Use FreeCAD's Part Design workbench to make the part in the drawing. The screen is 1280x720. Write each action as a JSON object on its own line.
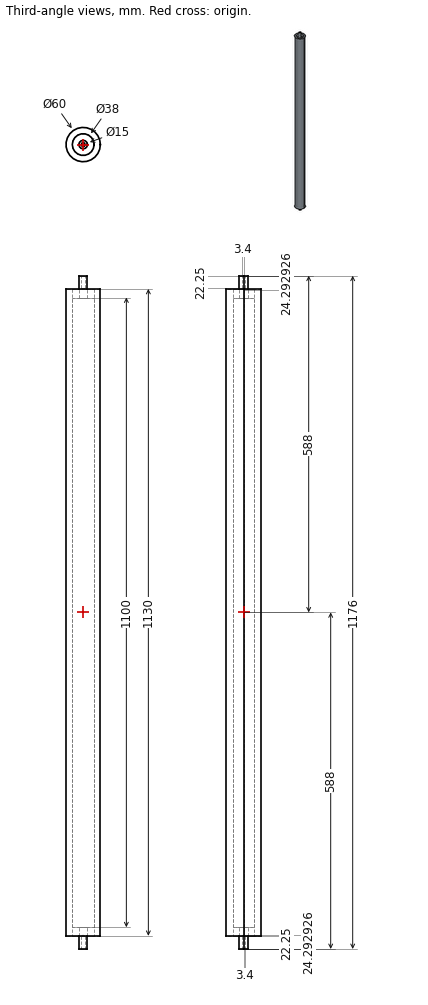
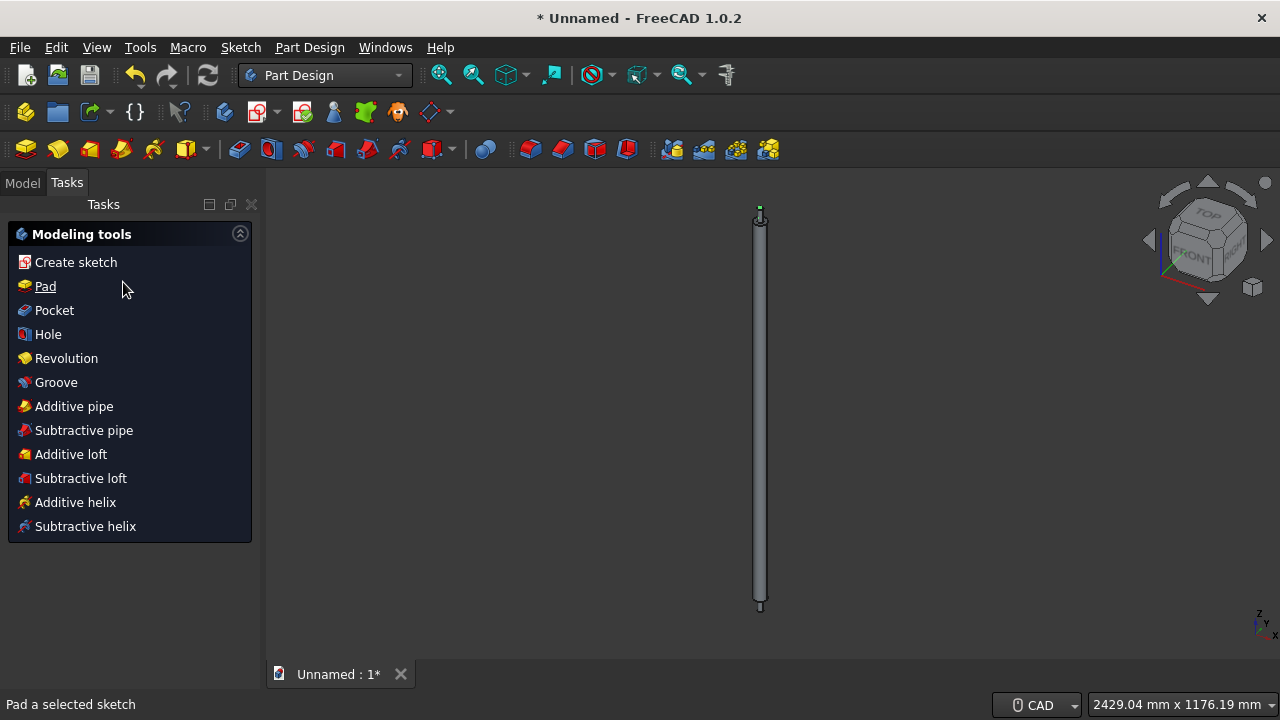
{"action": "left_click", "coordinate": [304, 150]}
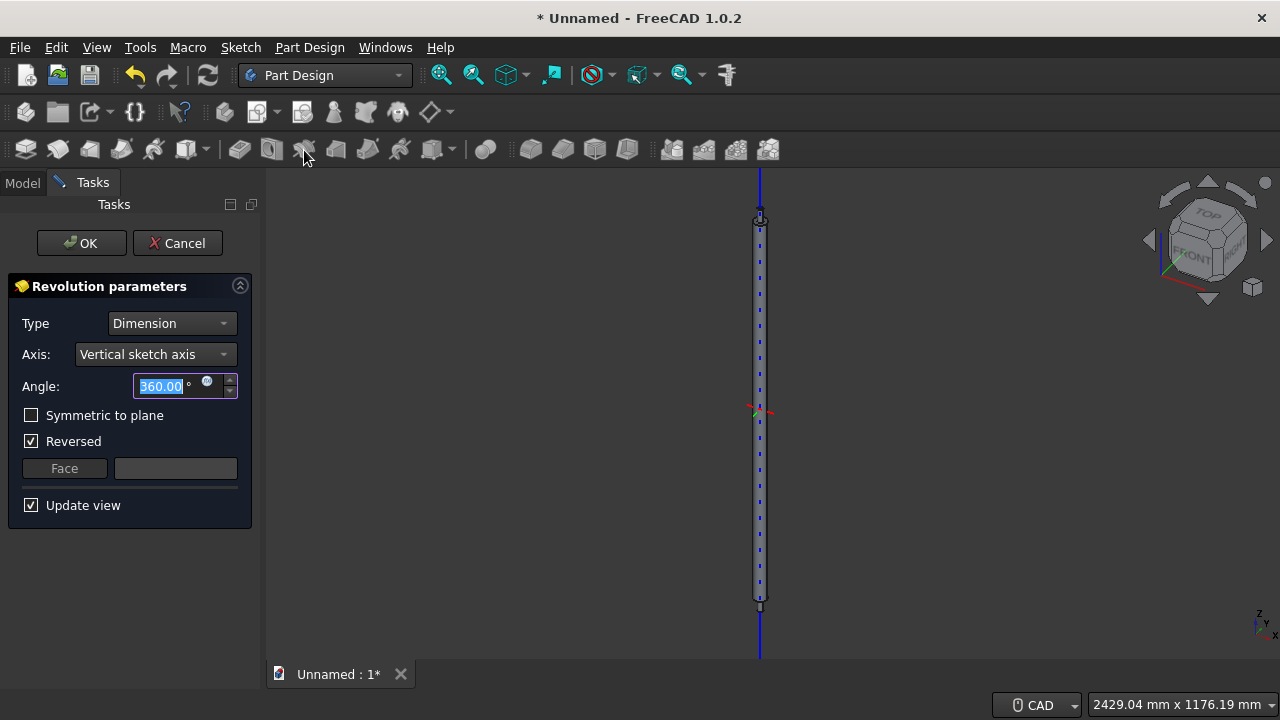
{"action": "left_click", "coordinate": [82, 243]}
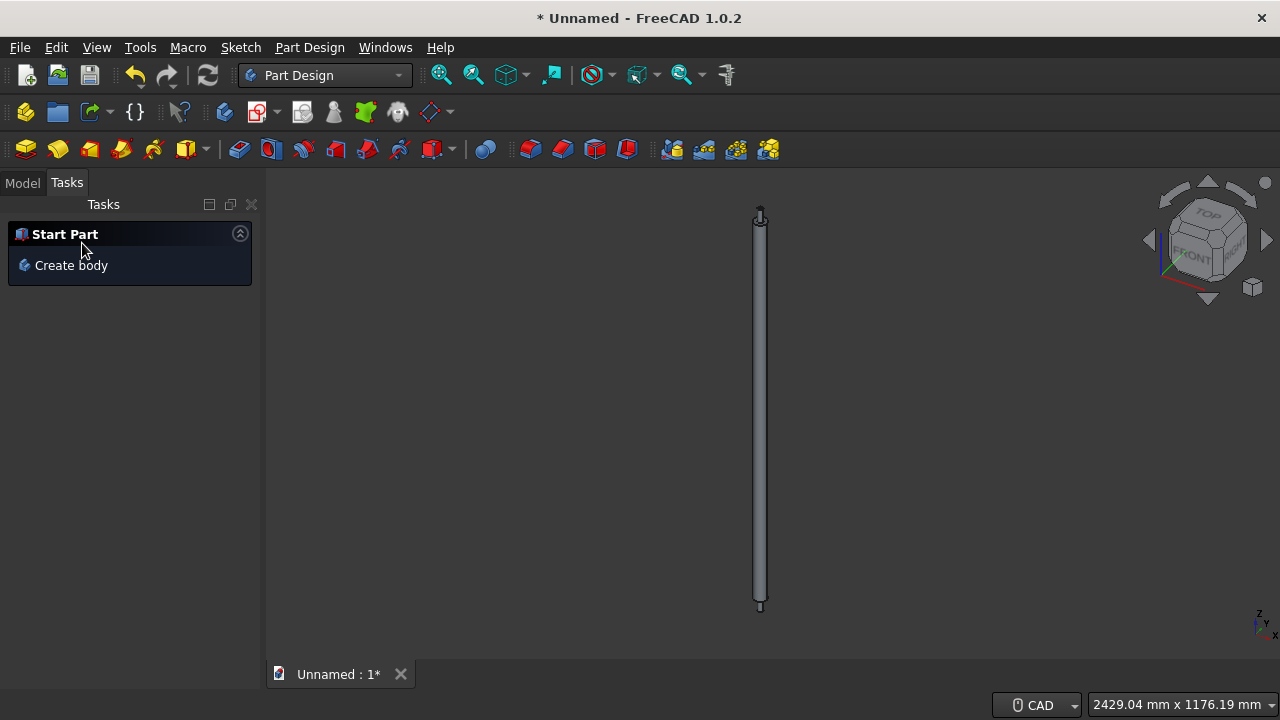
{"action": "left_click", "coordinate": [226, 112]}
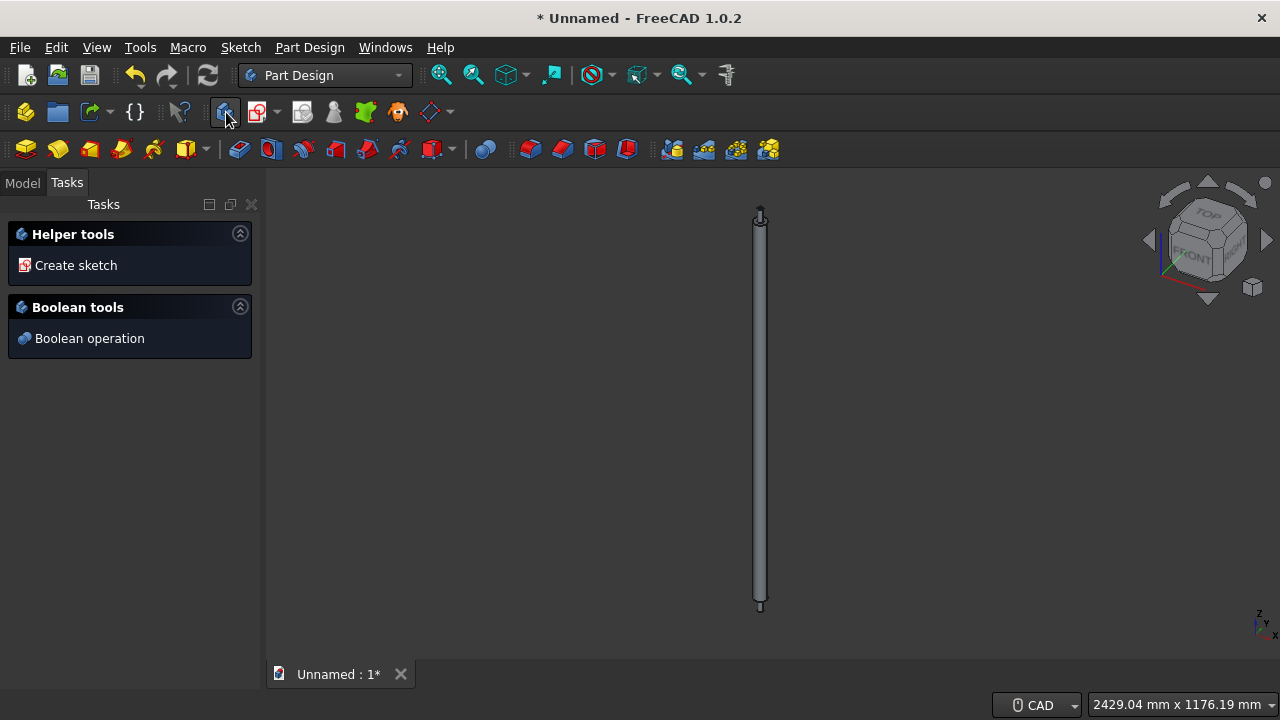
{"action": "left_click", "coordinate": [306, 619]}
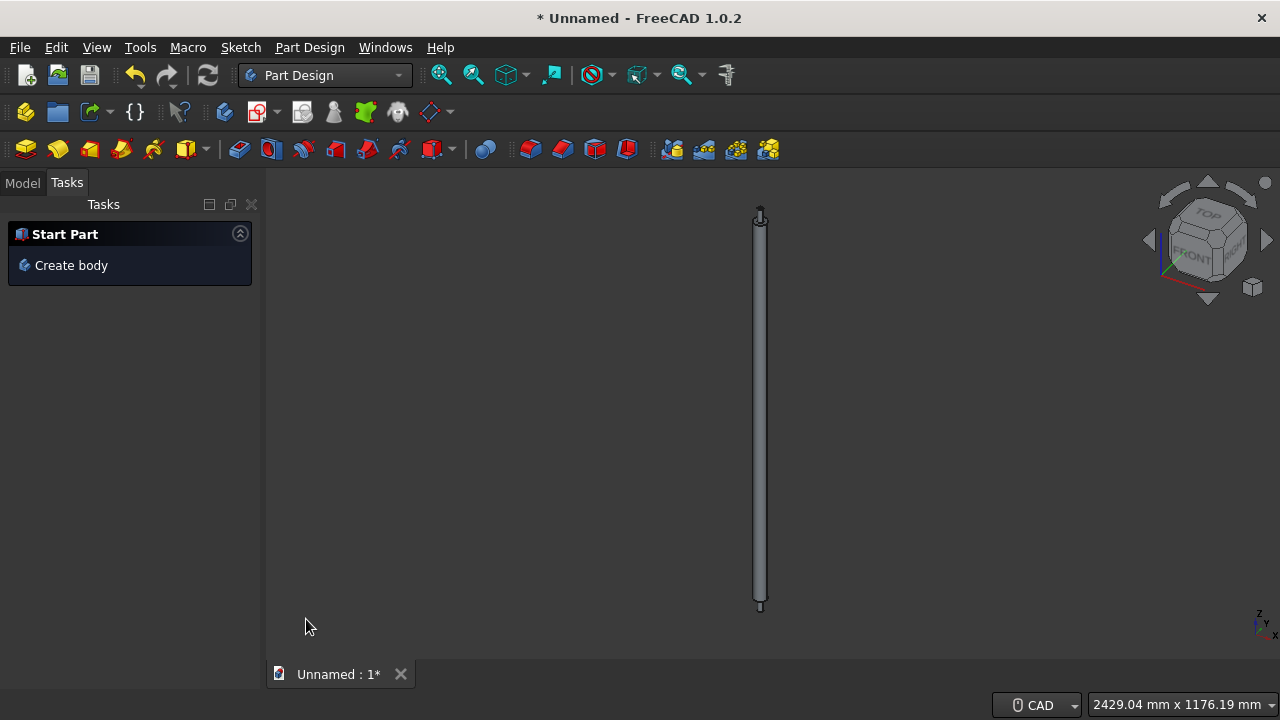
{"action": "left_click", "coordinate": [258, 112]}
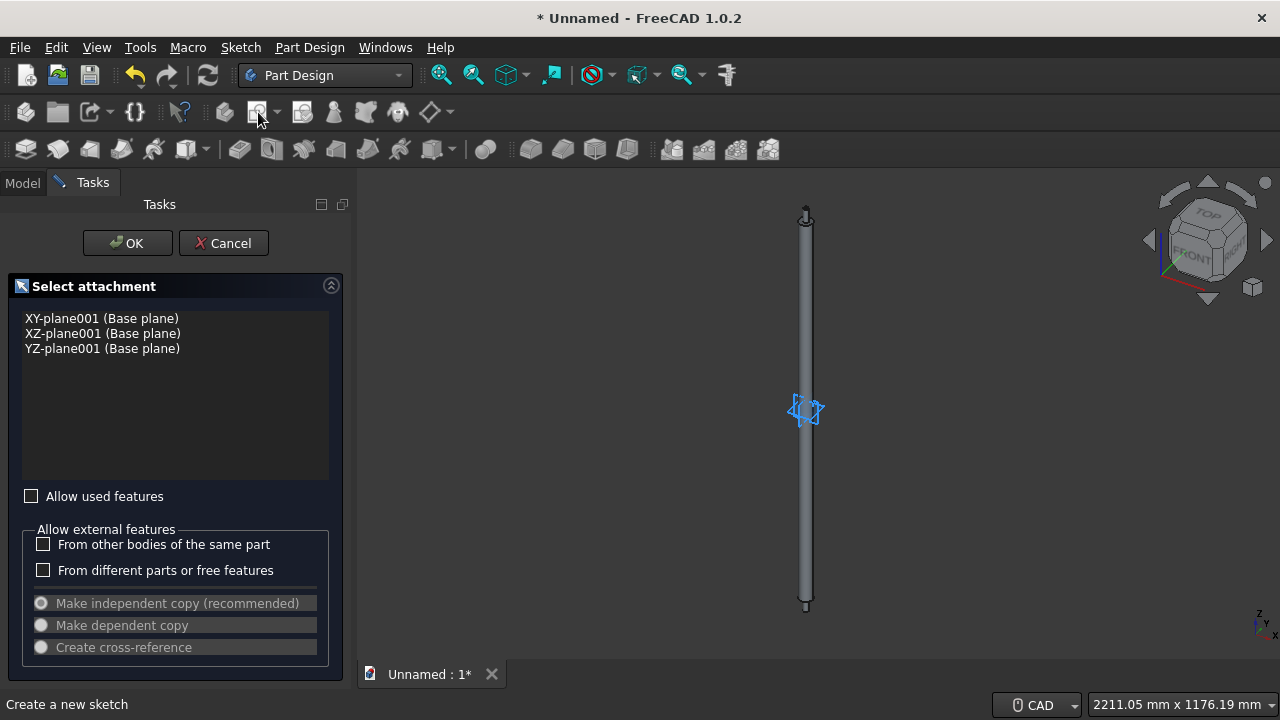
{"action": "left_click", "coordinate": [82, 318]}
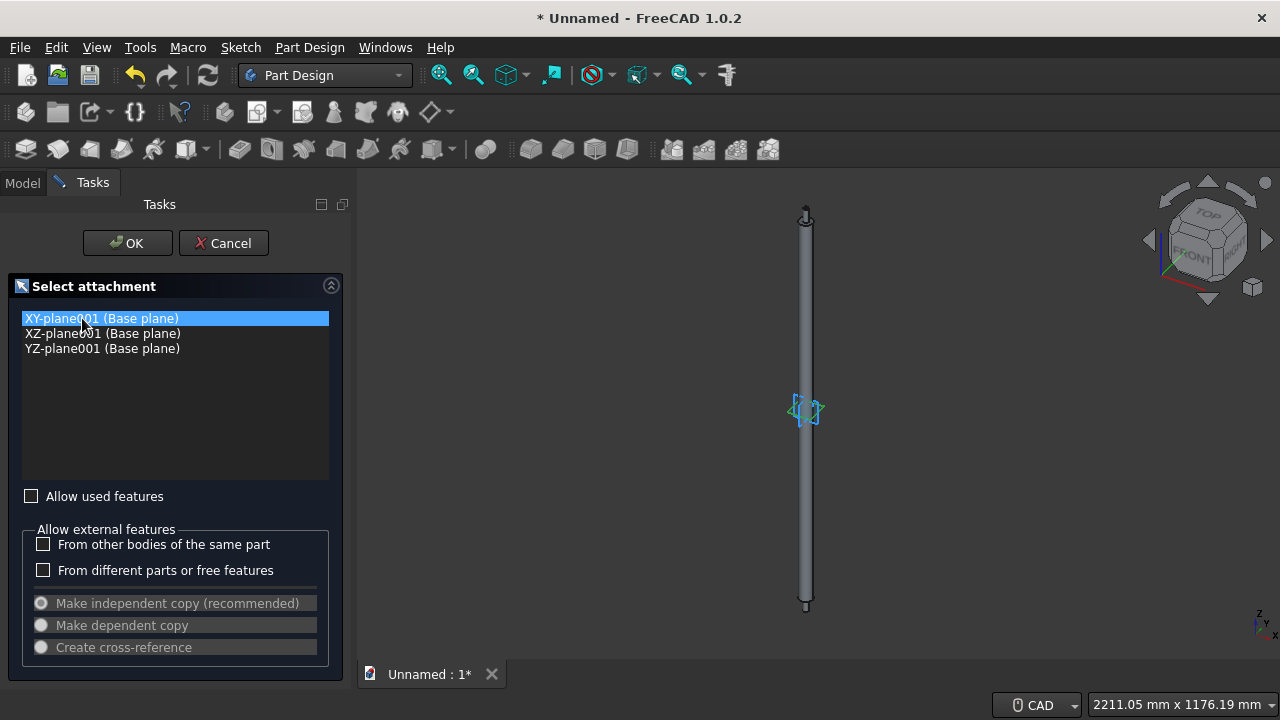
{"action": "left_click", "coordinate": [128, 243]}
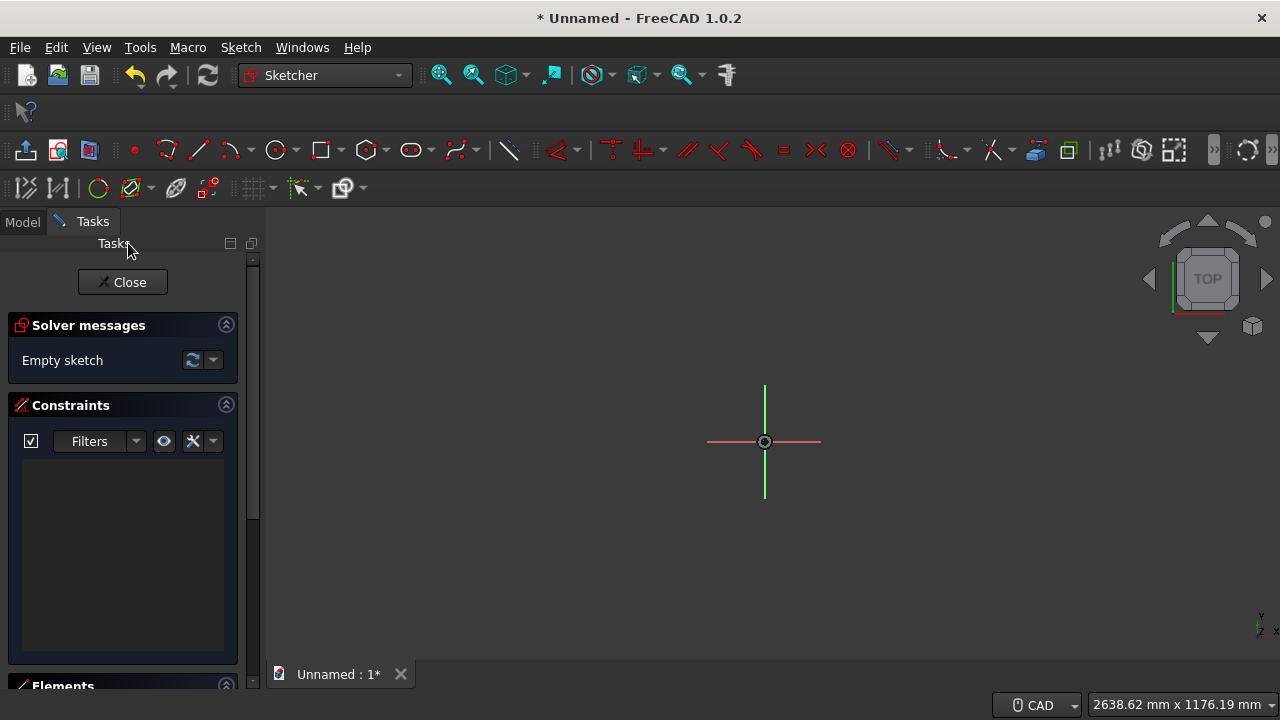
{"action": "scroll", "coordinate": [771, 443], "scroll_direction": "up", "scroll_amount": 12}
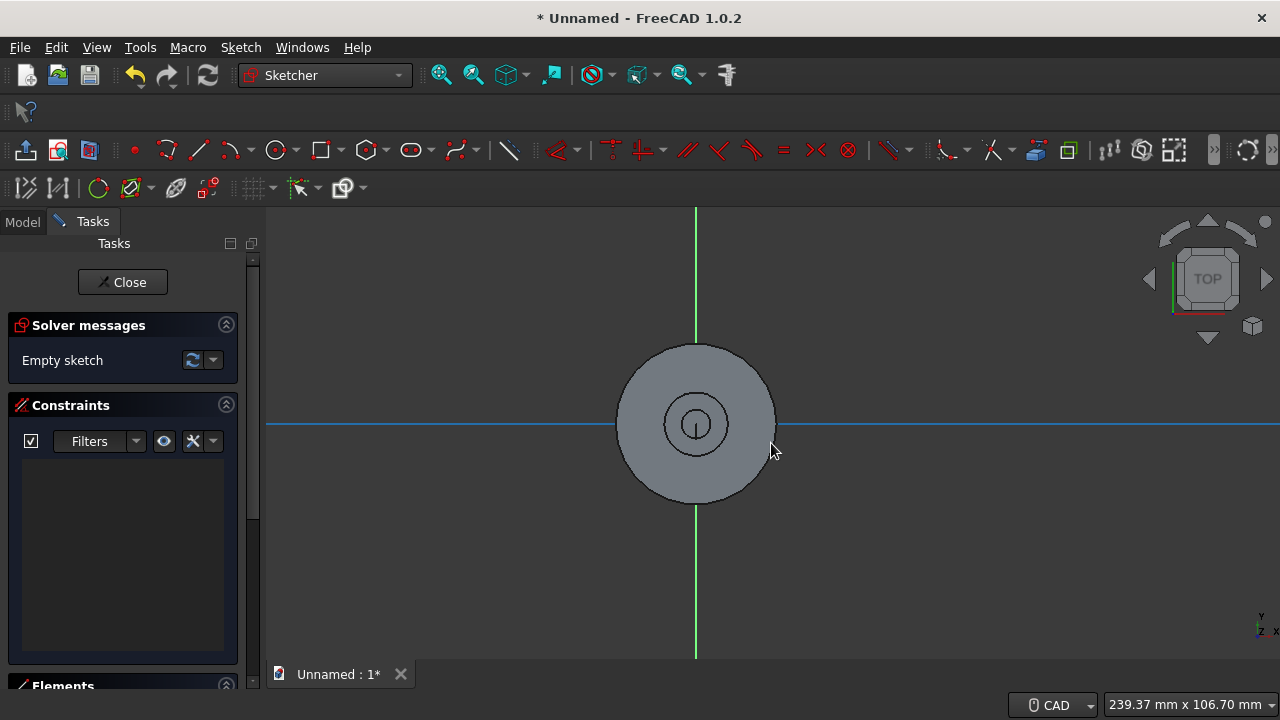
{"action": "left_click", "coordinate": [276, 150]}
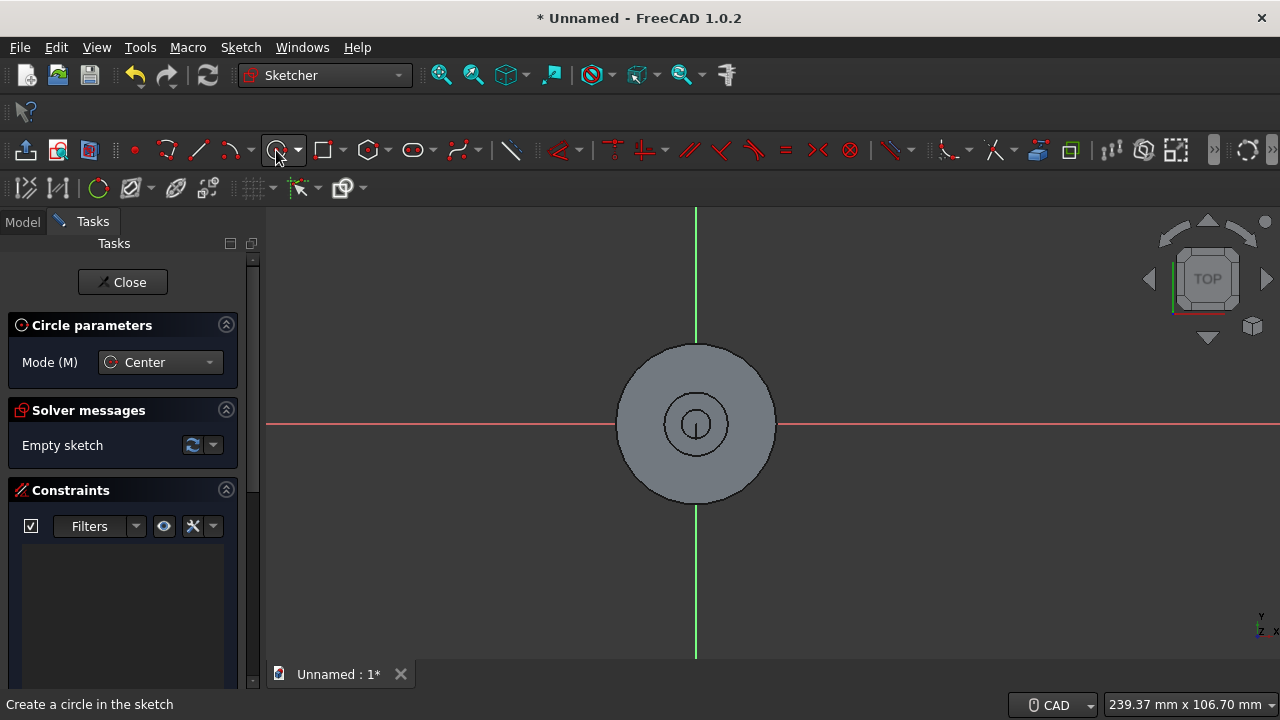
{"action": "left_click", "coordinate": [696, 424]}
{"action": "left_click", "coordinate": [786, 334]}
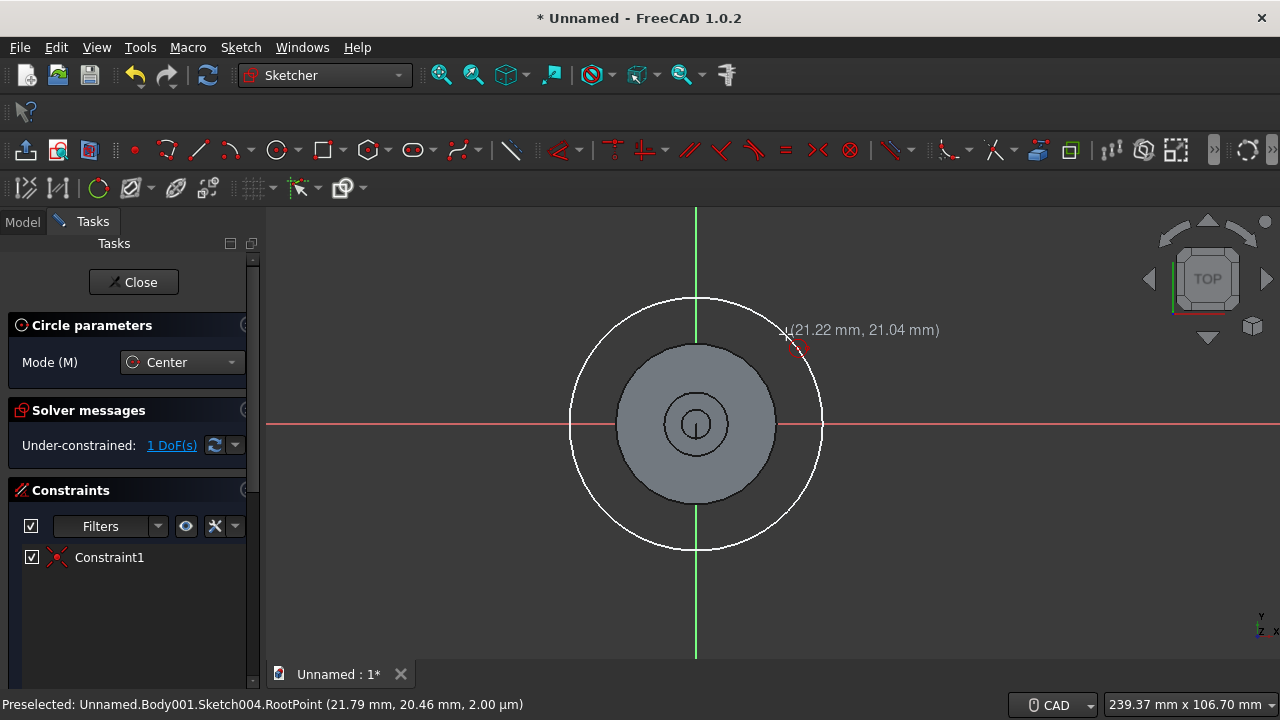
{"action": "left_click", "coordinate": [696, 424]}
{"action": "left_click", "coordinate": [753, 367]}
{"action": "key", "text": "Escape"}